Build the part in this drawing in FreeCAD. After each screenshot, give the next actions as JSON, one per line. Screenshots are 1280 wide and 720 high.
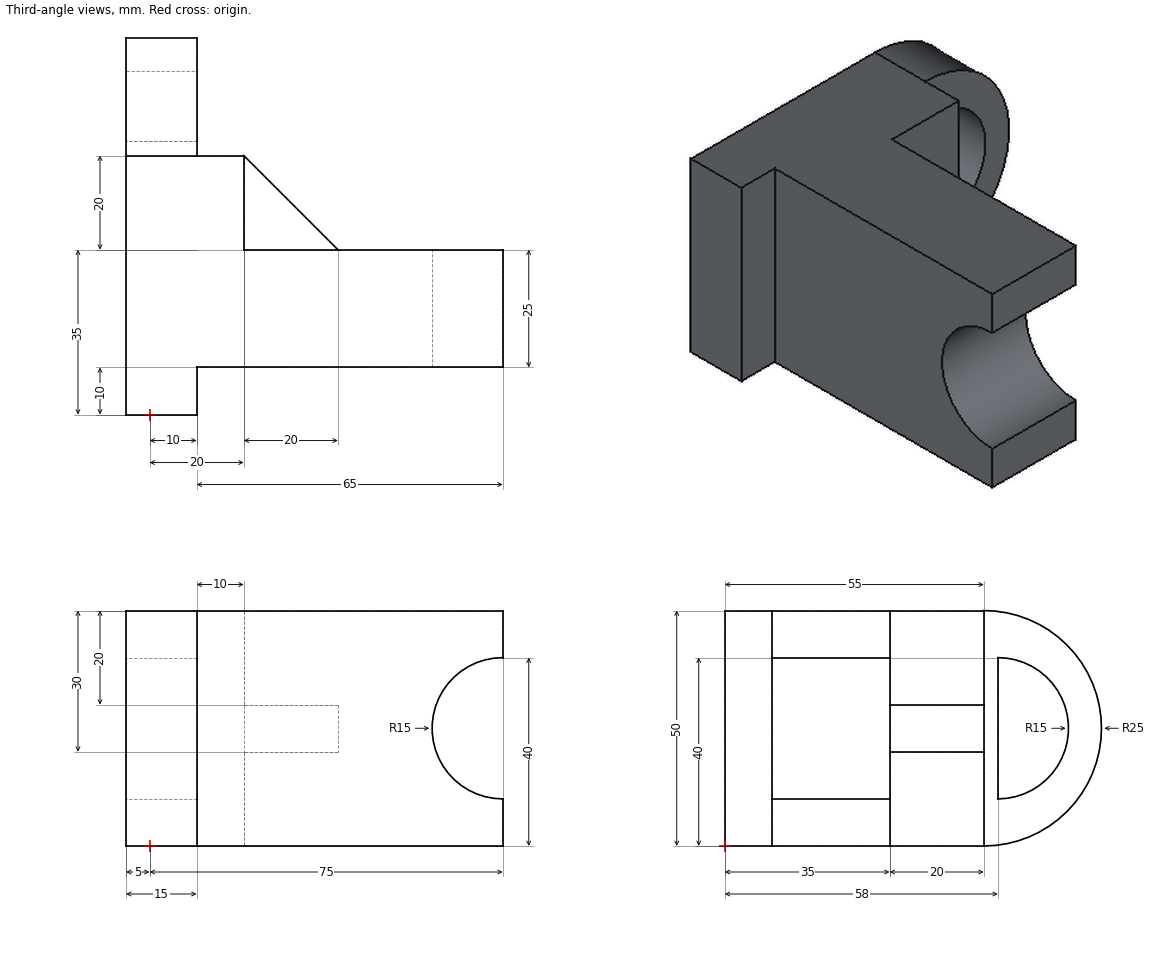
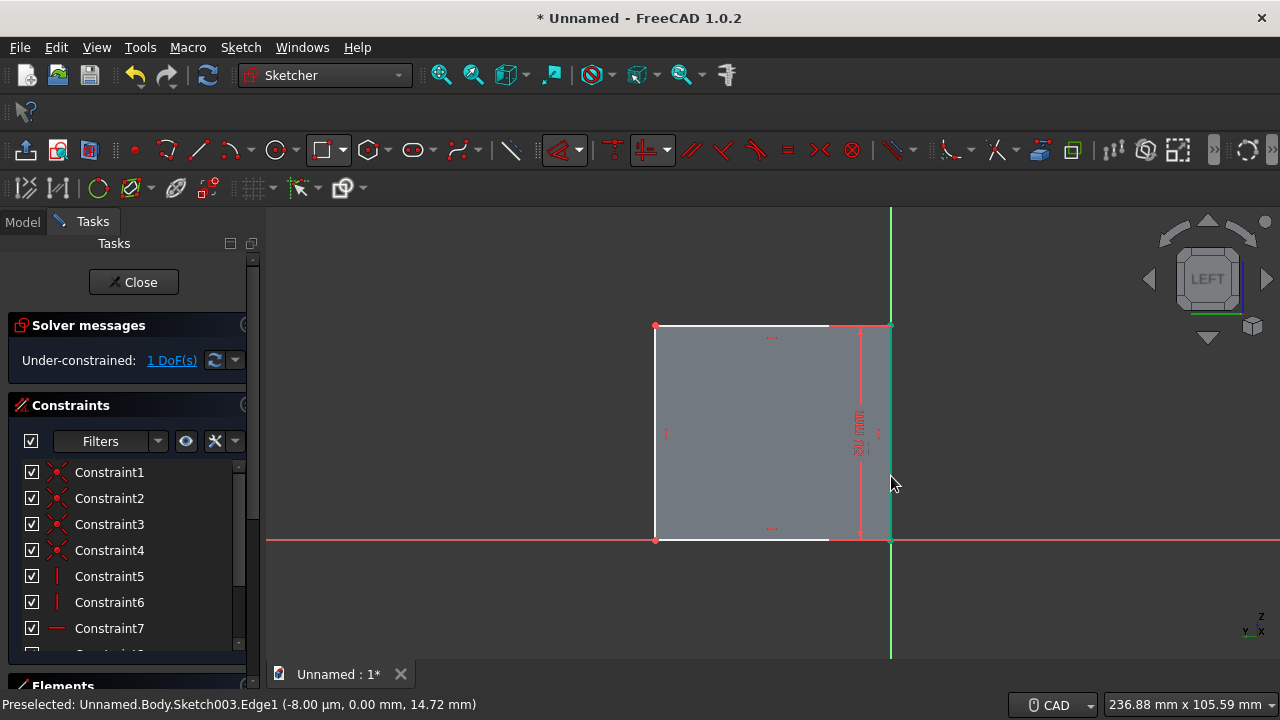
{"action": "left_click", "coordinate": [820, 326]}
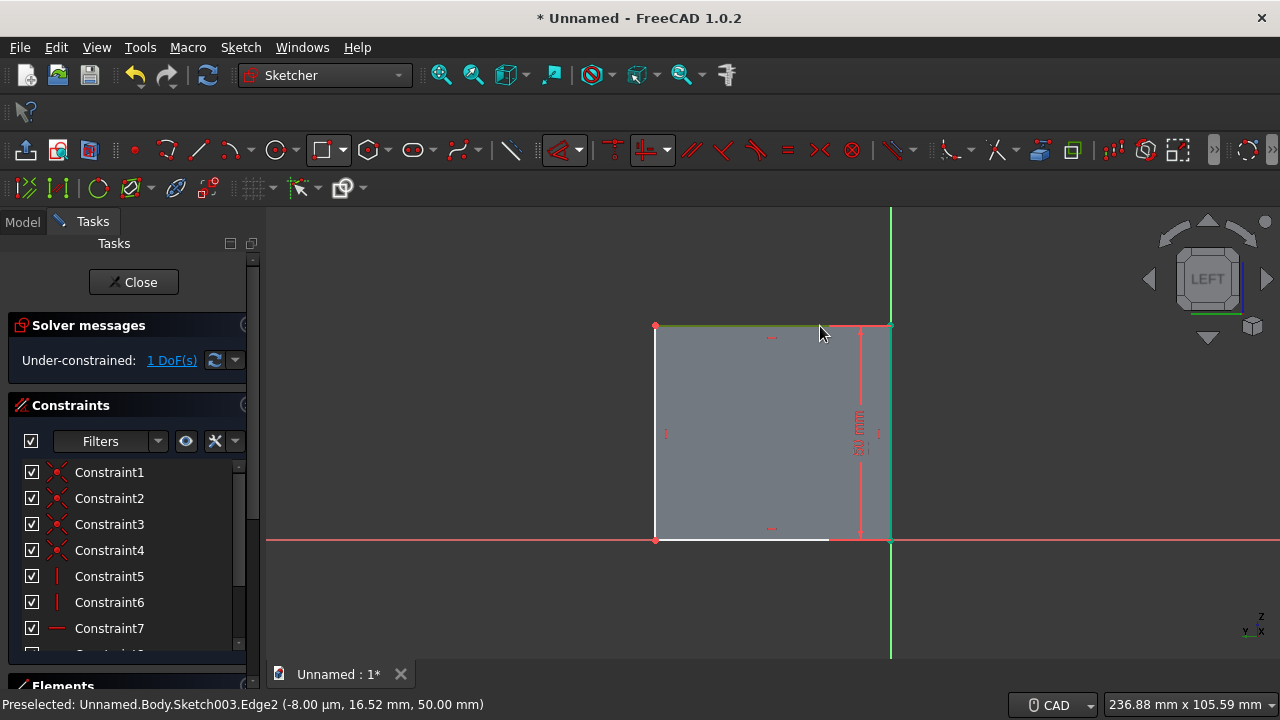
{"action": "left_click", "coordinate": [582, 150]}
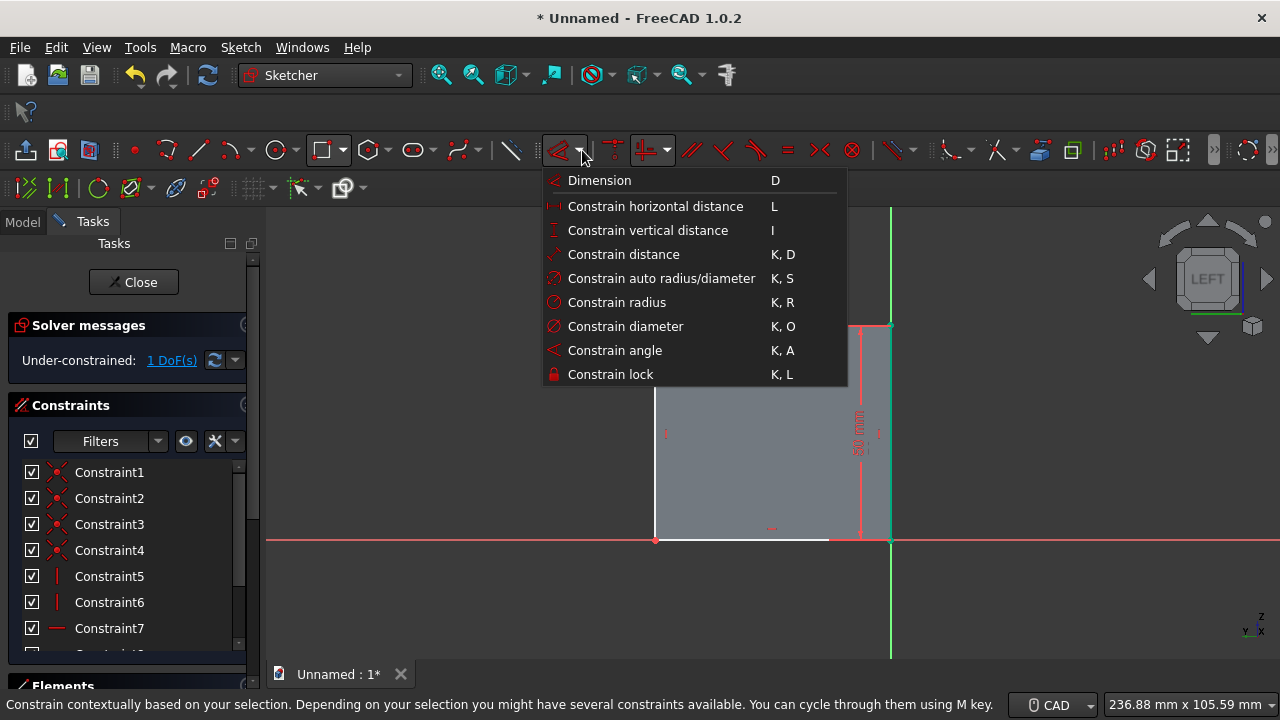
{"action": "left_click", "coordinate": [695, 206]}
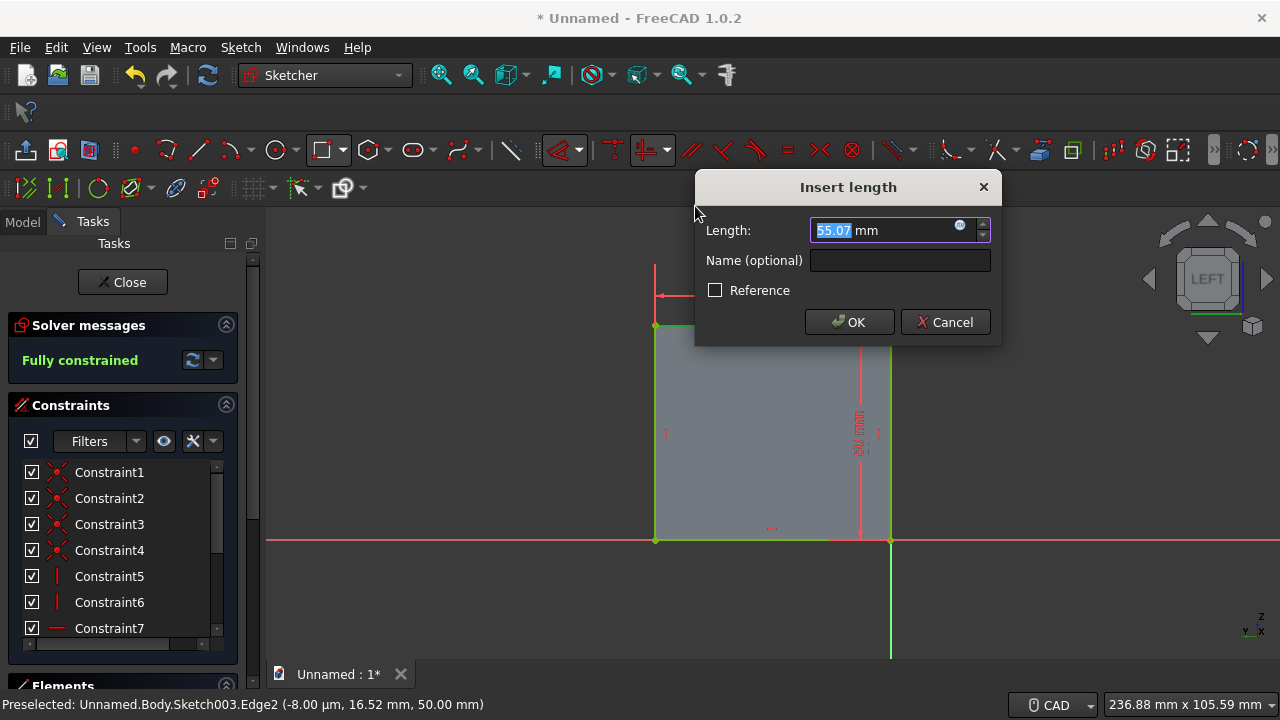
{"action": "type", "text": "55"}
{"action": "key", "text": "Return"}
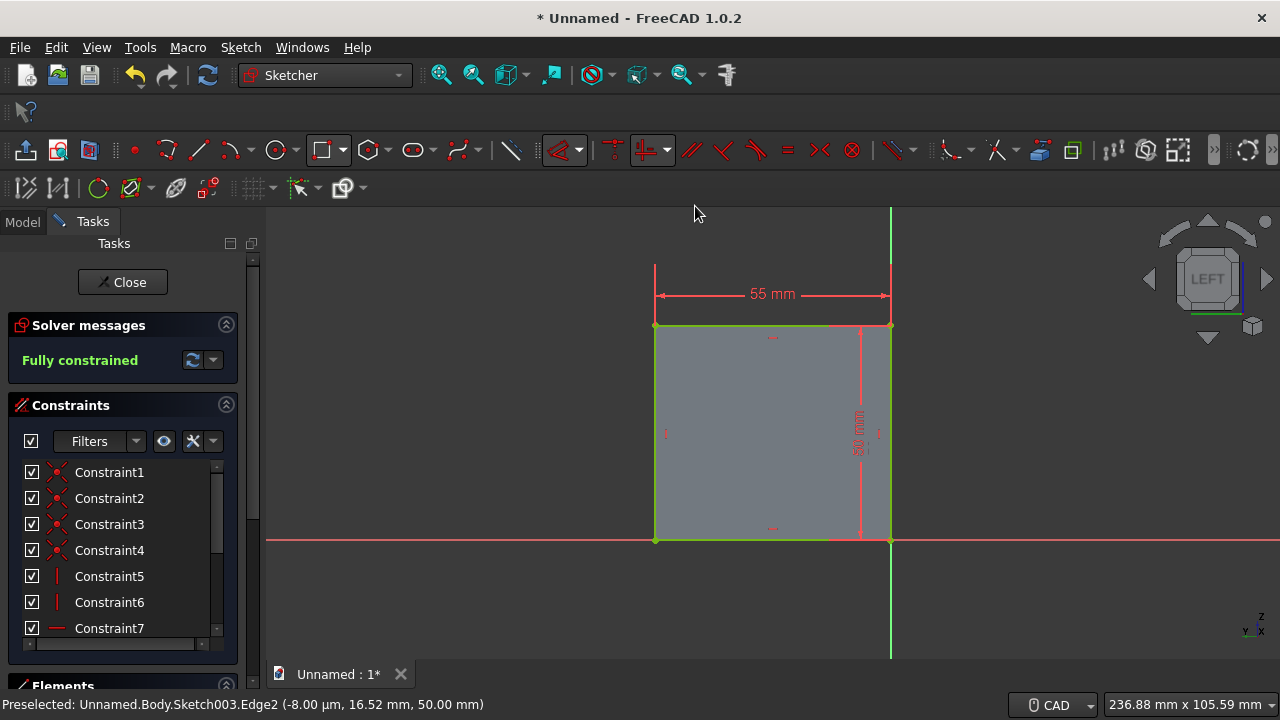
{"action": "left_click", "coordinate": [123, 282]}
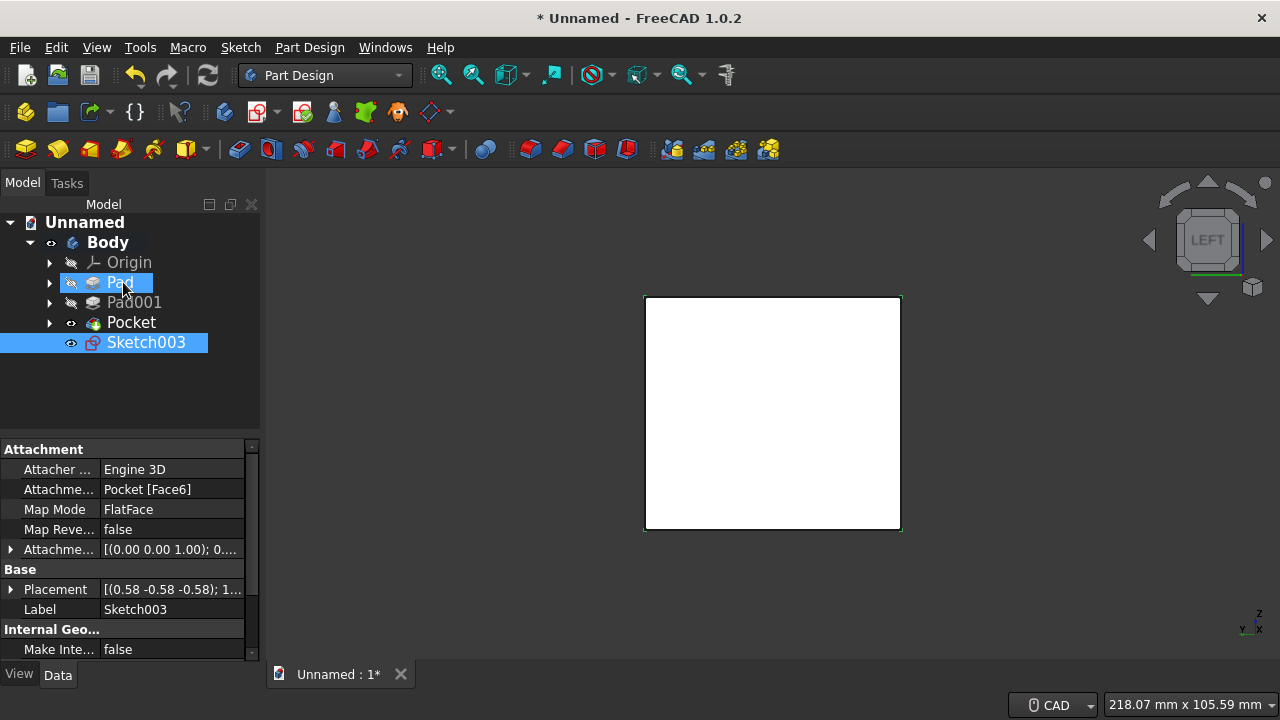
{"action": "left_click", "coordinate": [26, 150]}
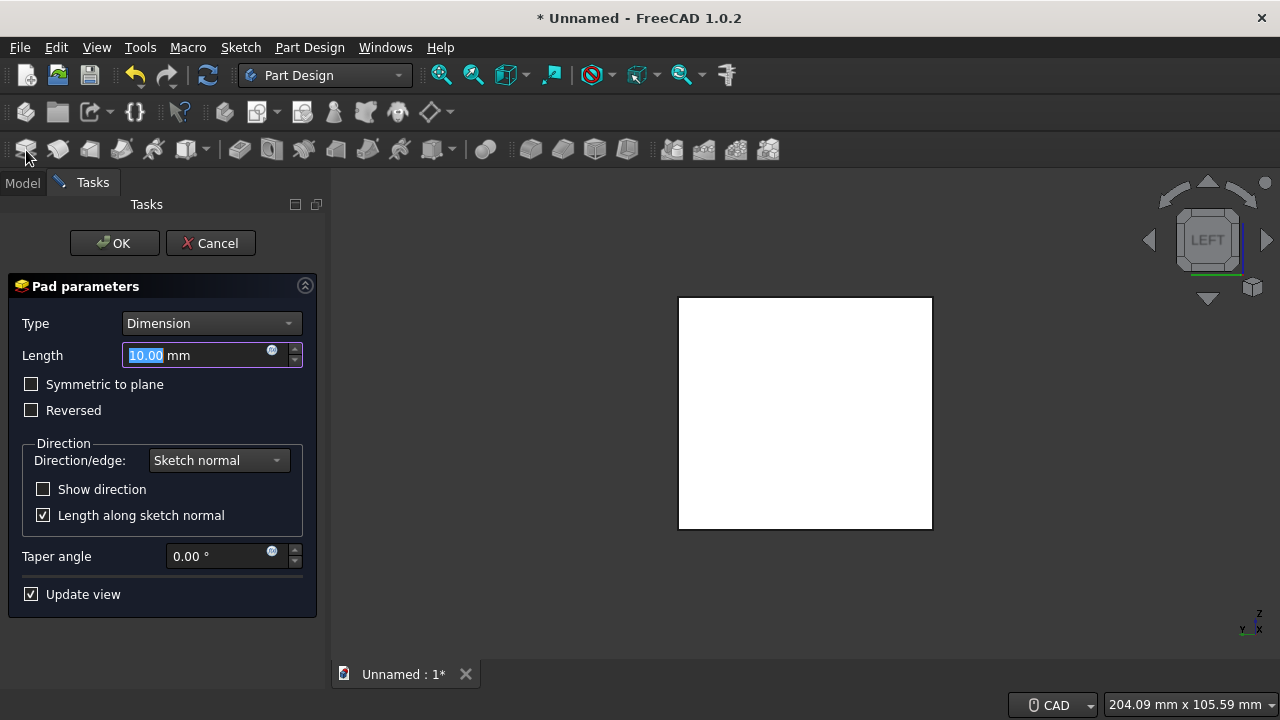
{"action": "type", "text": "5"}
{"action": "key", "text": "Tab"}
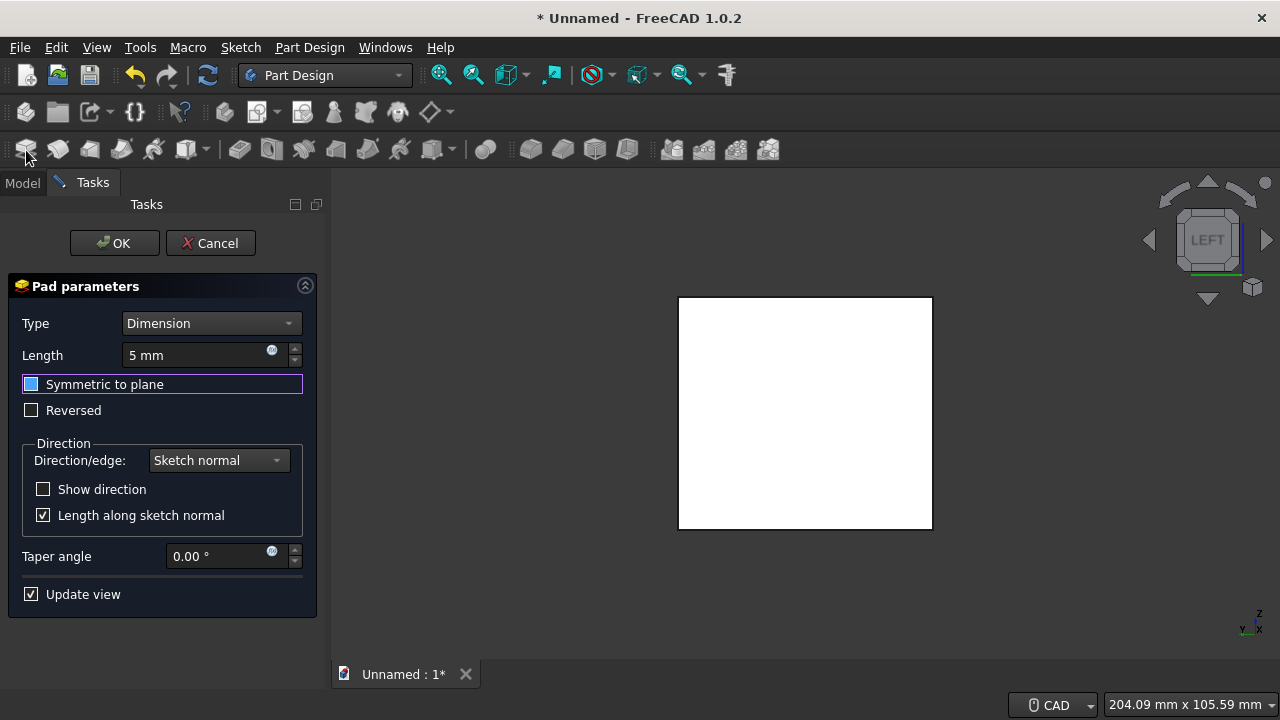
{"action": "left_click", "coordinate": [115, 243]}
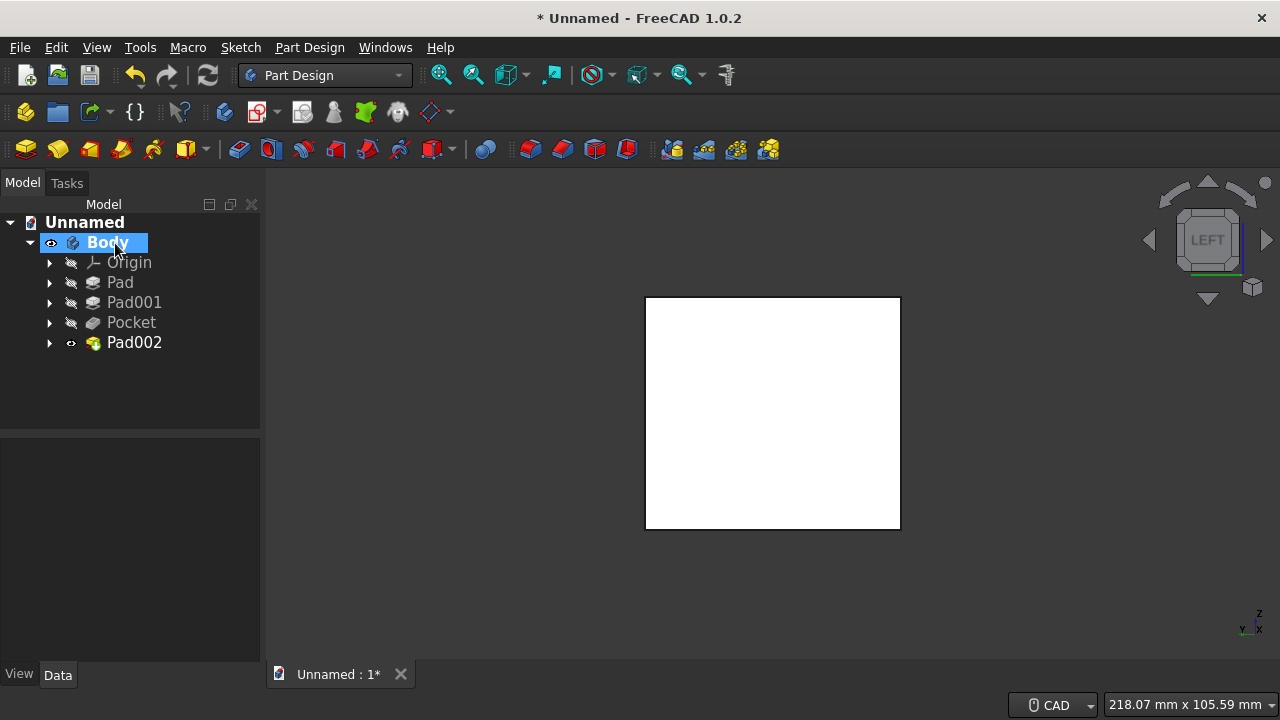
{"action": "left_click", "coordinate": [773, 413]}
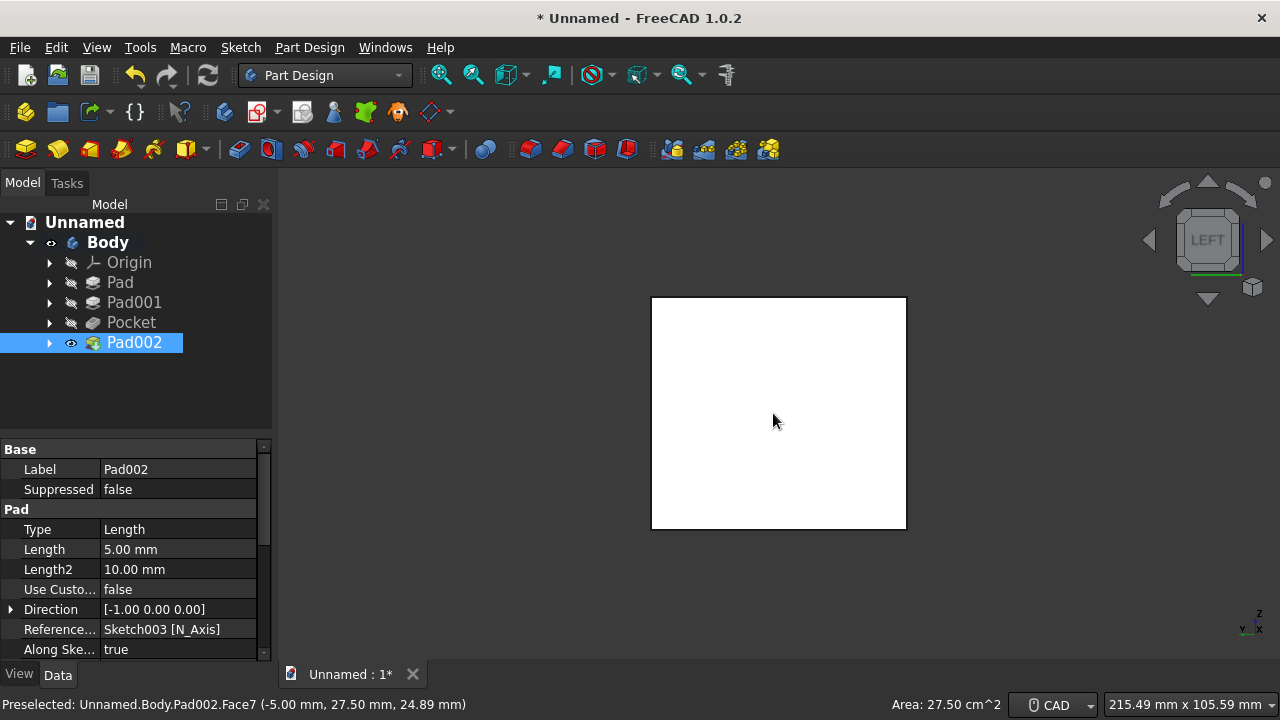
{"action": "left_click", "coordinate": [258, 112]}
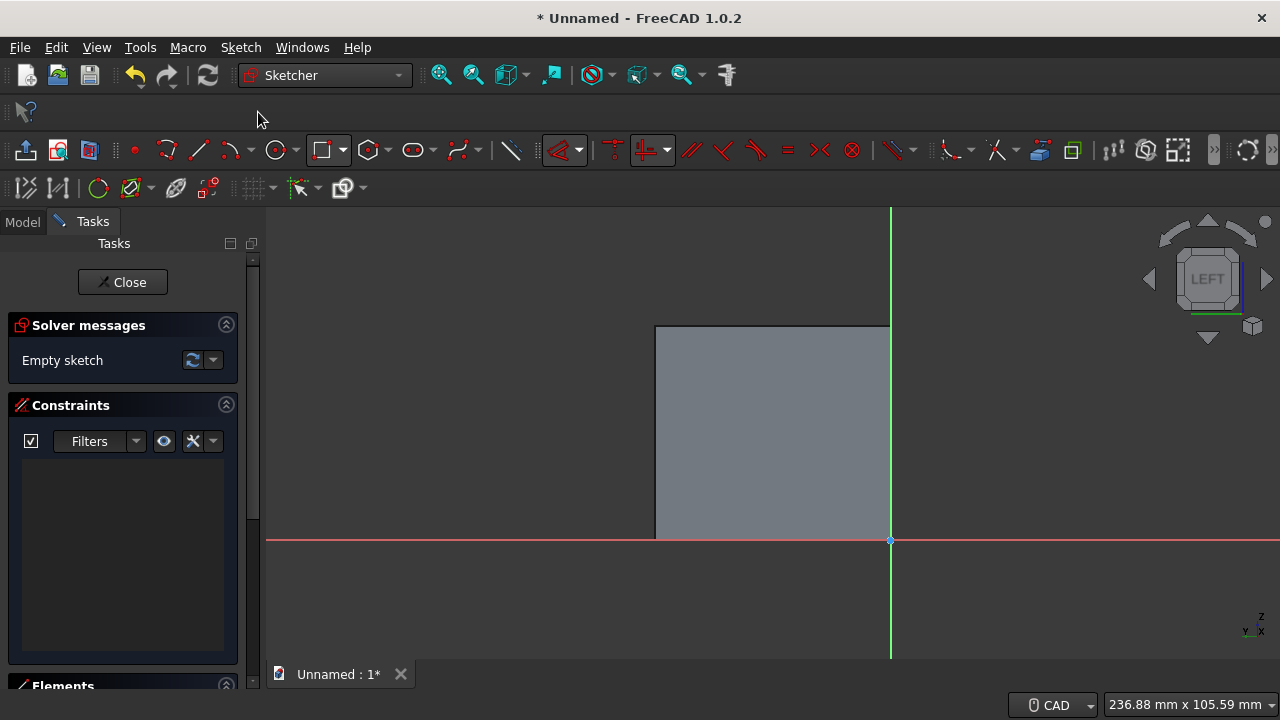
{"action": "left_click", "coordinate": [200, 150]}